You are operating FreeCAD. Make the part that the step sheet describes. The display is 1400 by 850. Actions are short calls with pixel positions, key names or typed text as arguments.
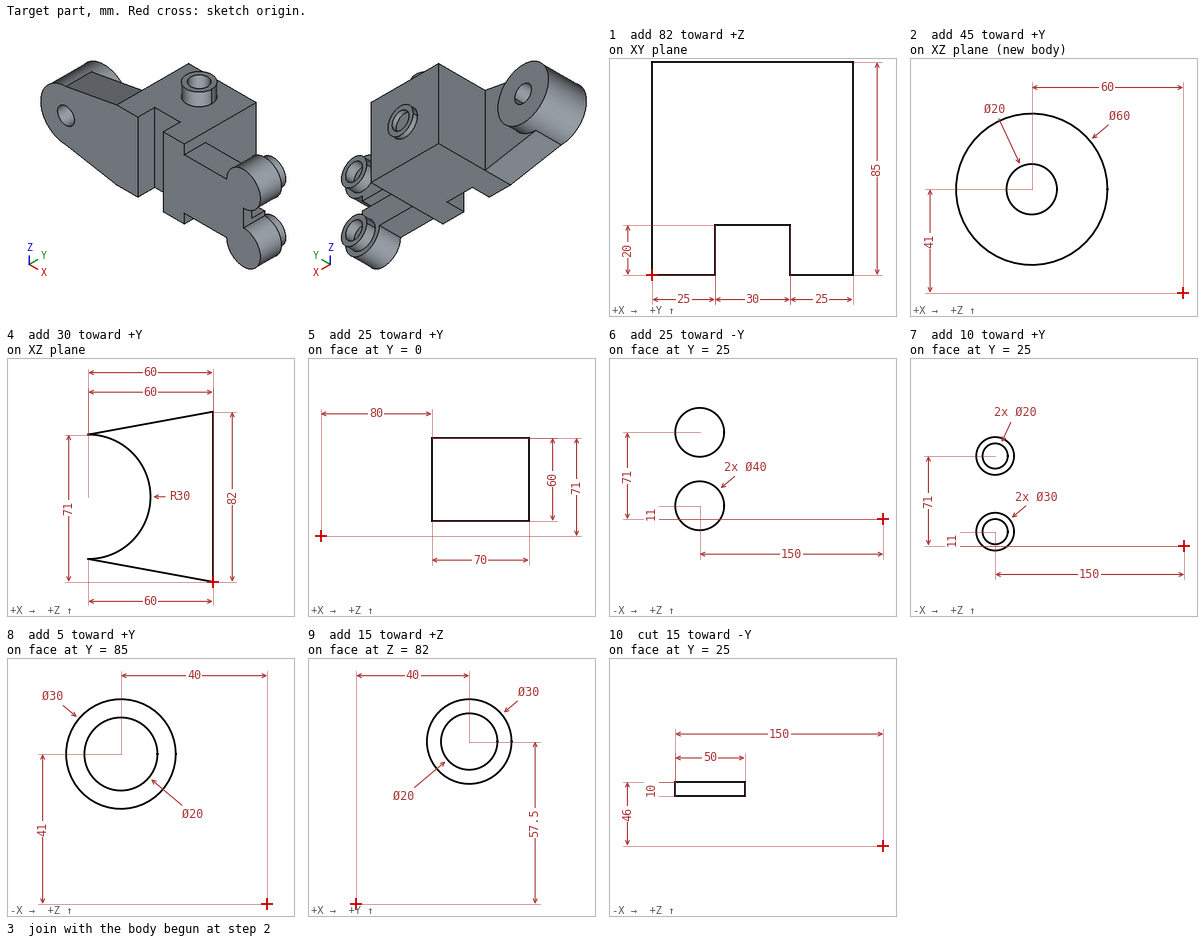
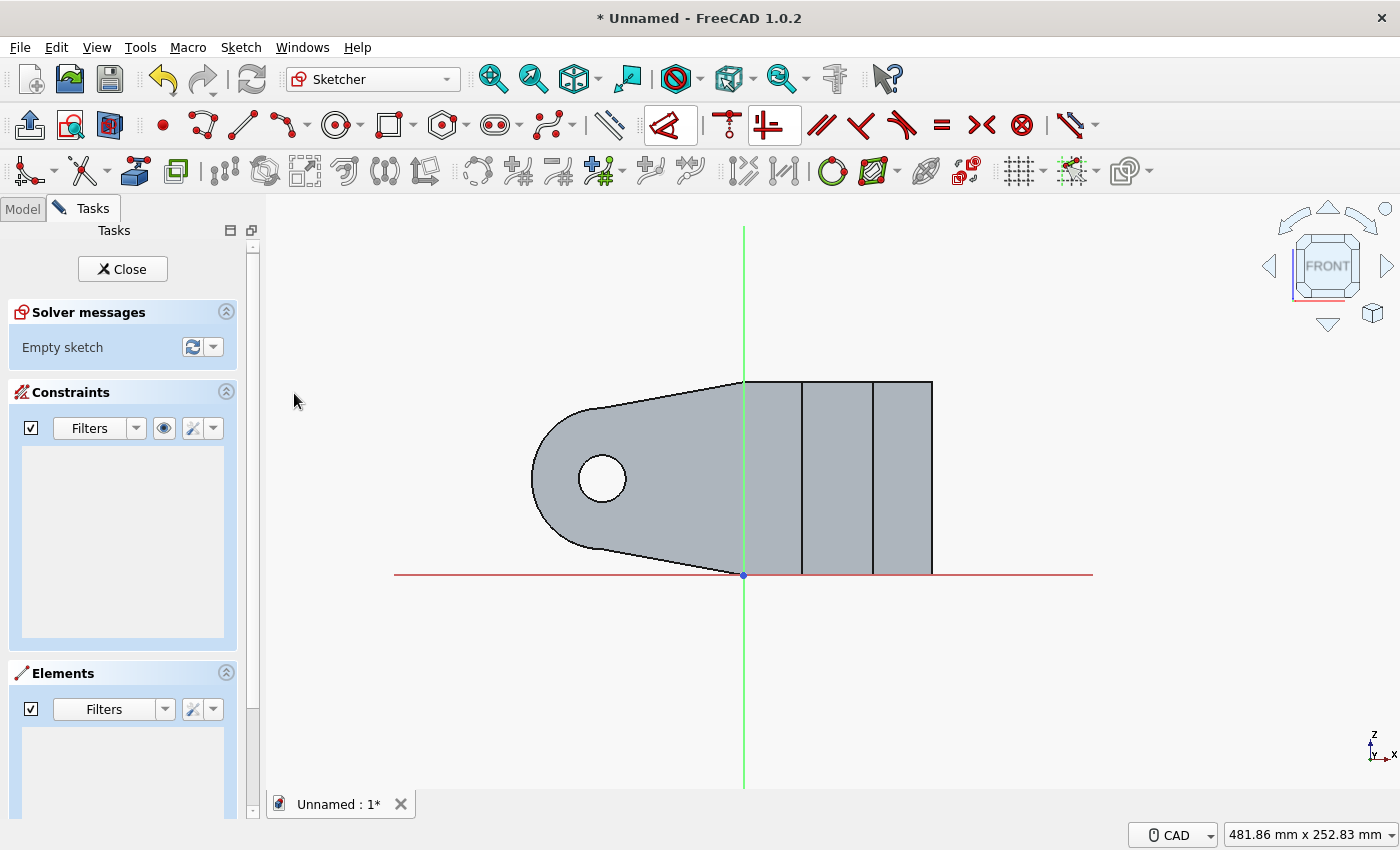
scroll(1109, 492, up, 3)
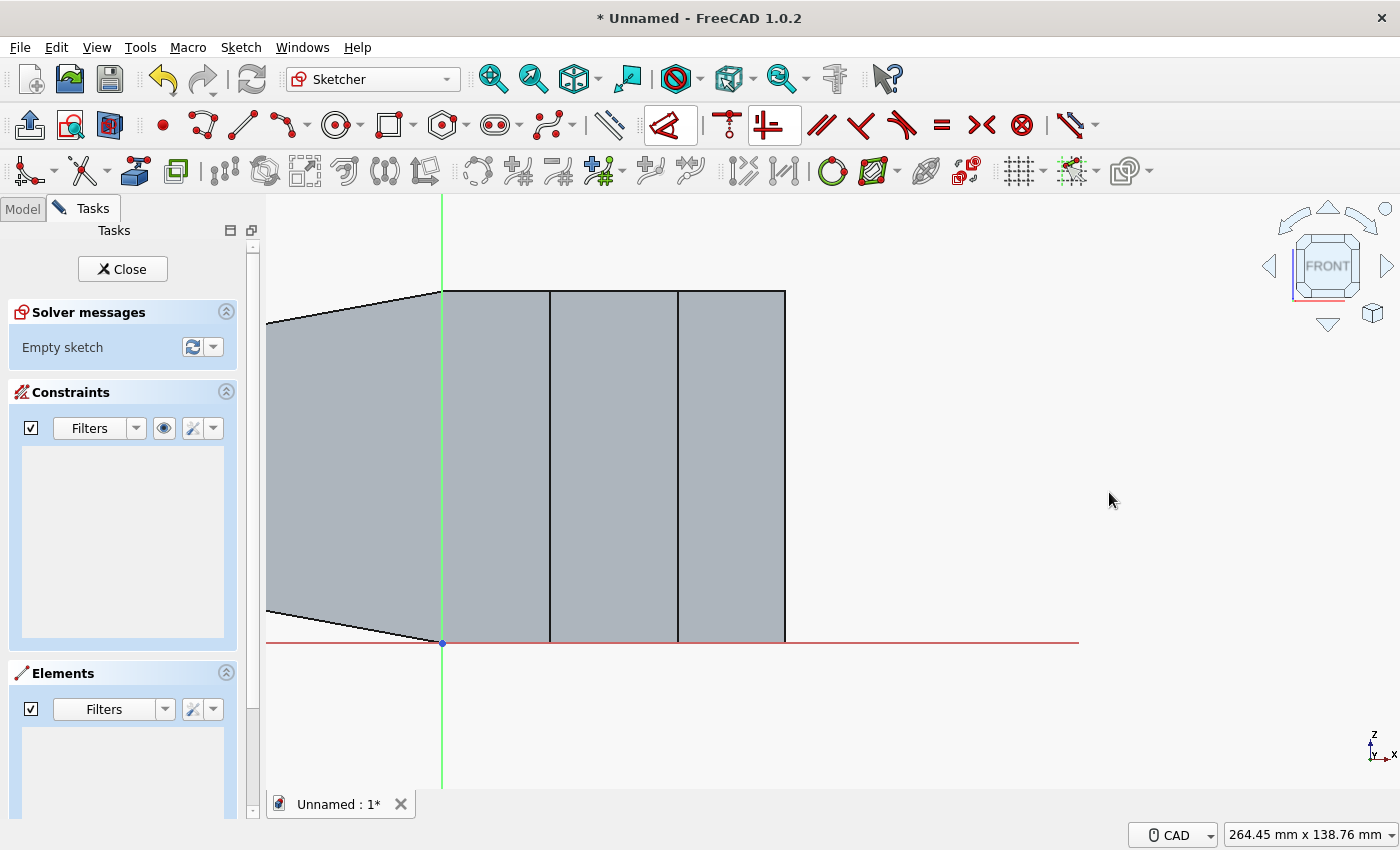
click(390, 126)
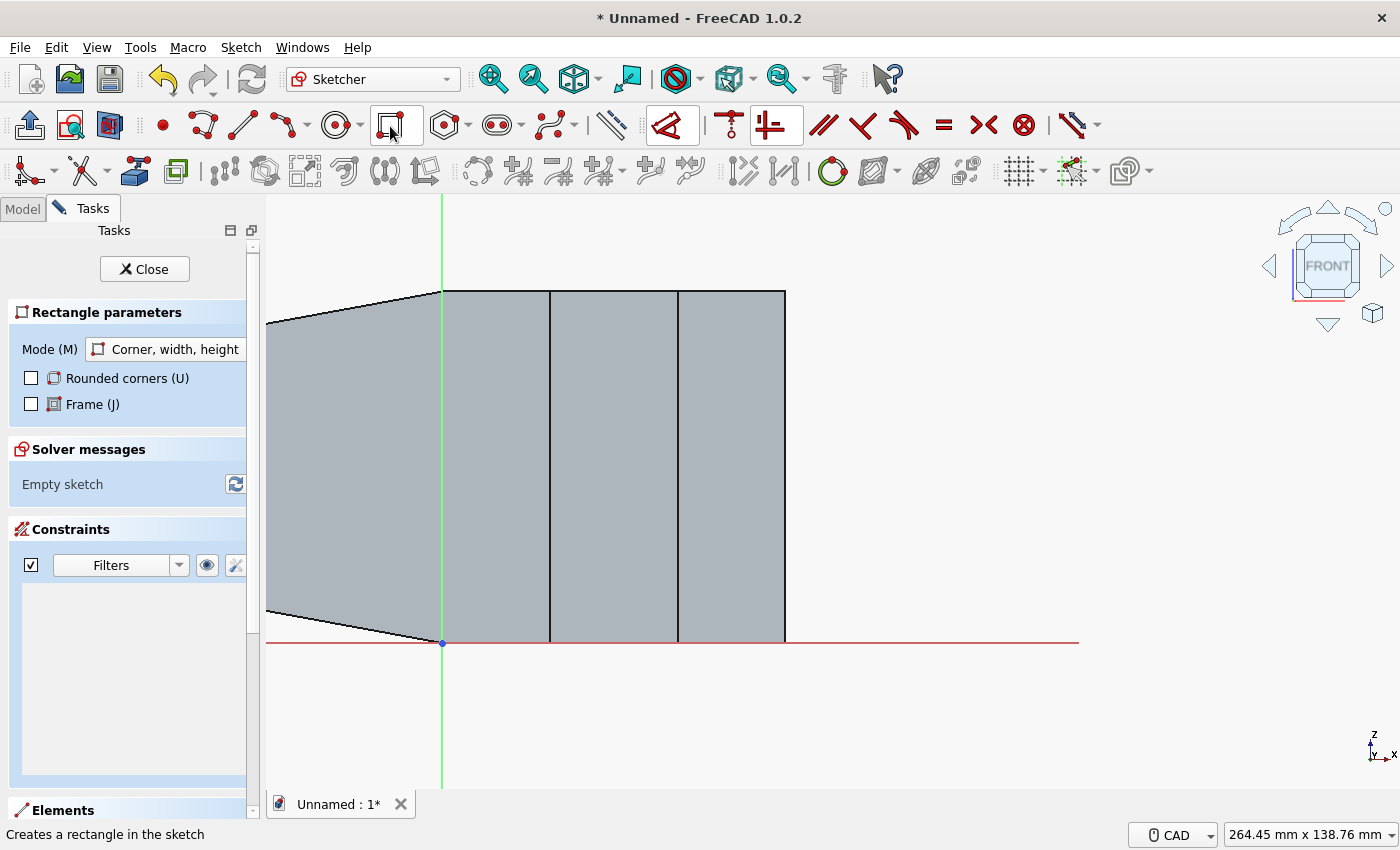
click(785, 339)
click(1086, 596)
key(Escape)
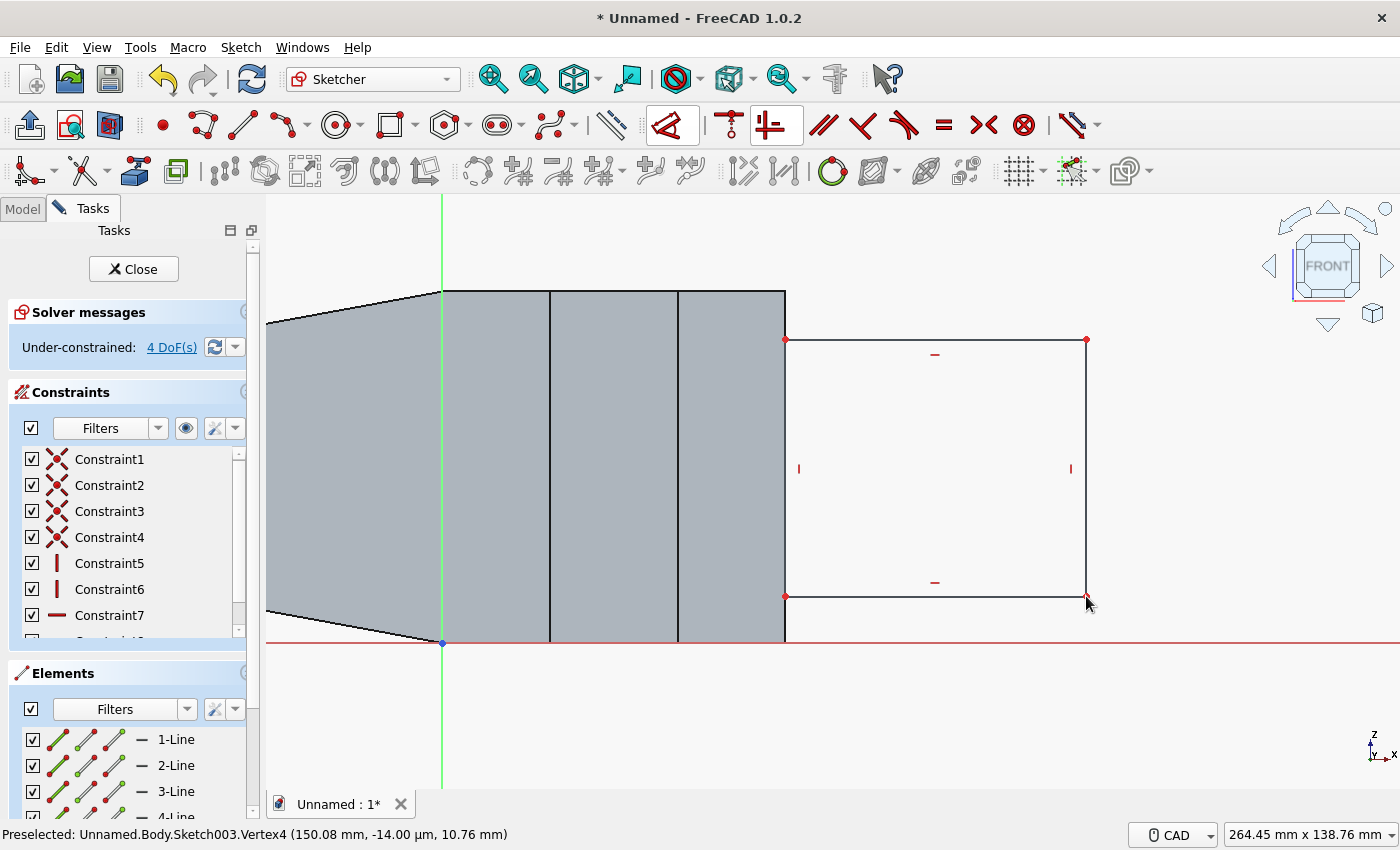
click(785, 417)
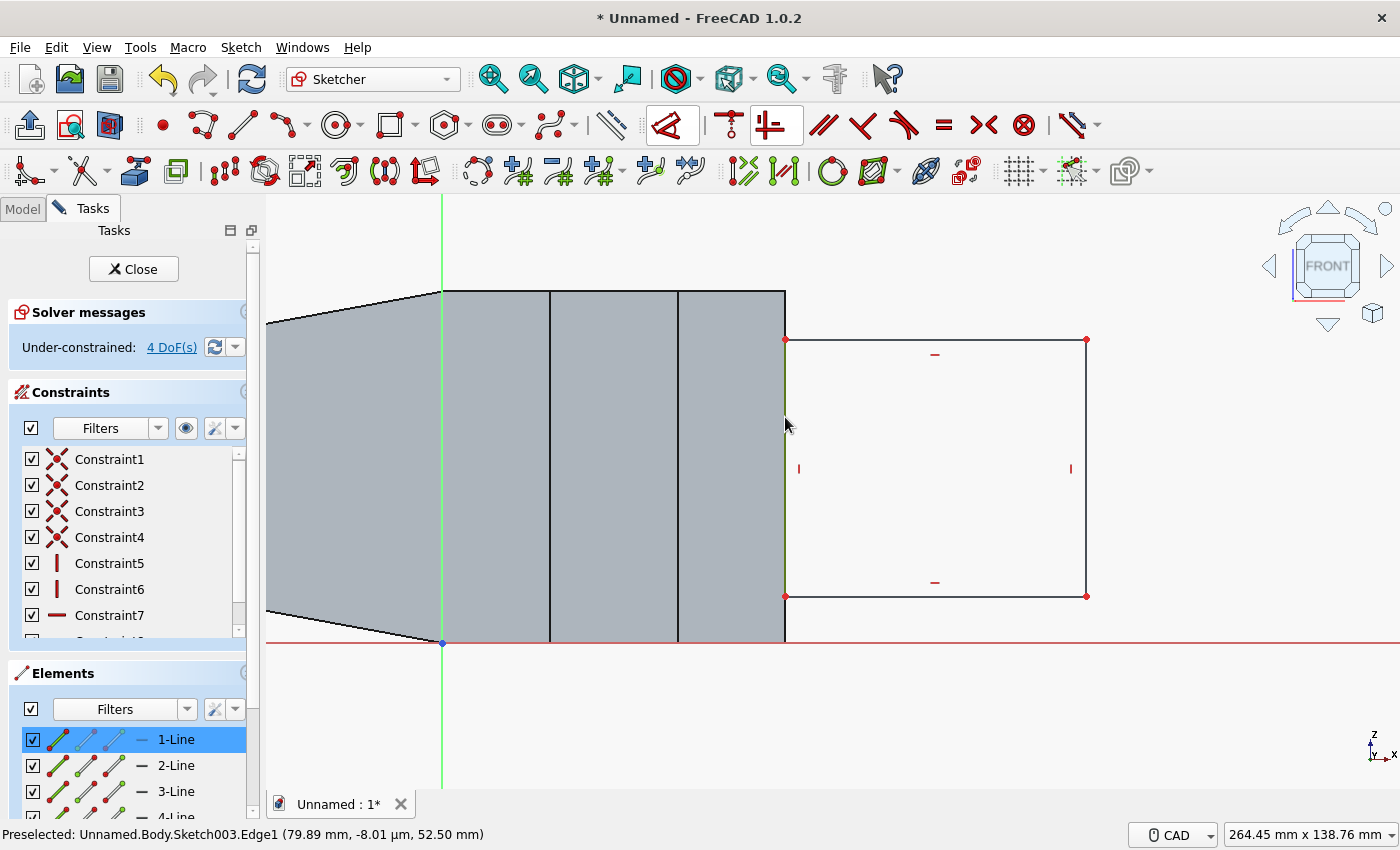
key(i)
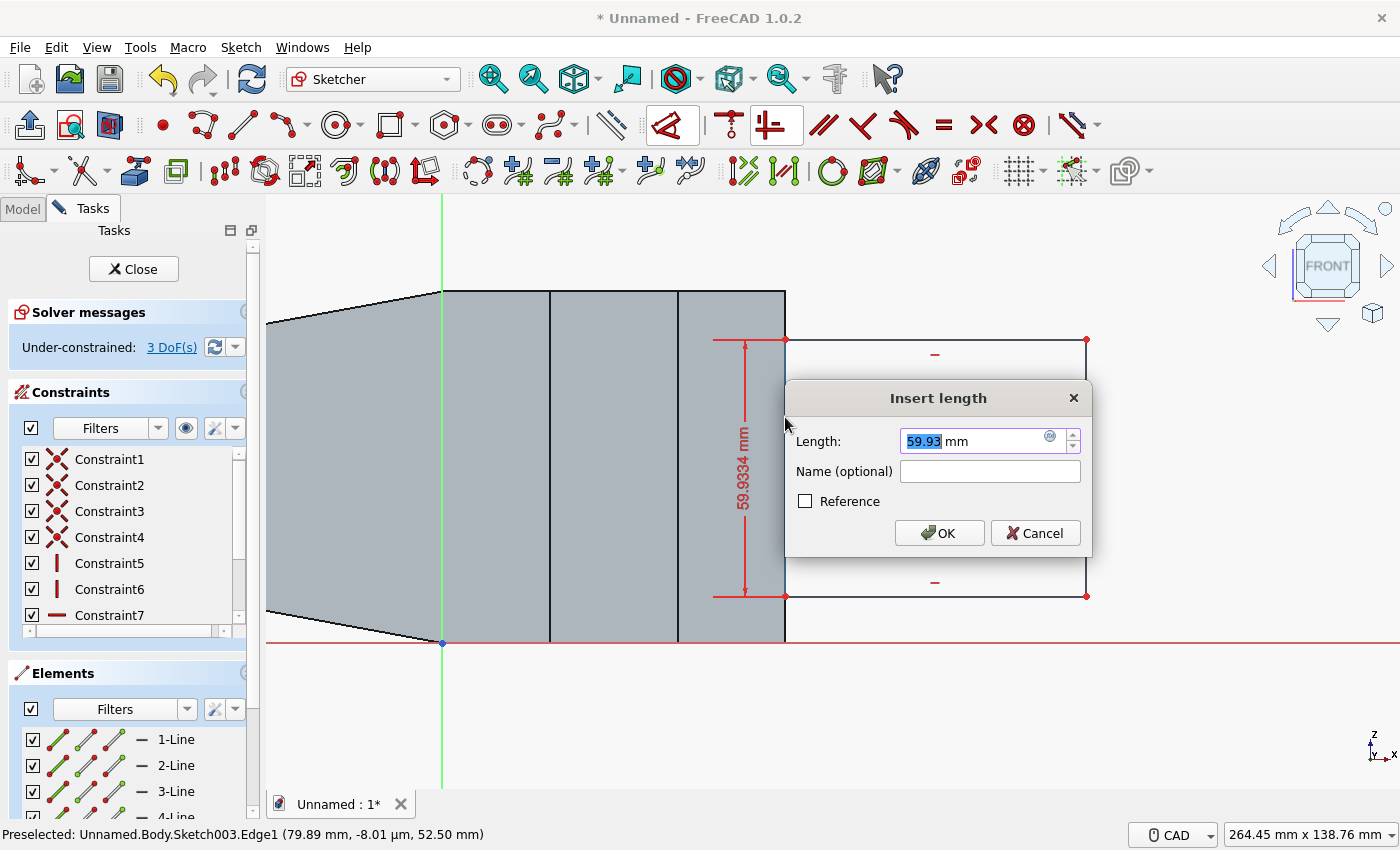
text(60)
key(Return)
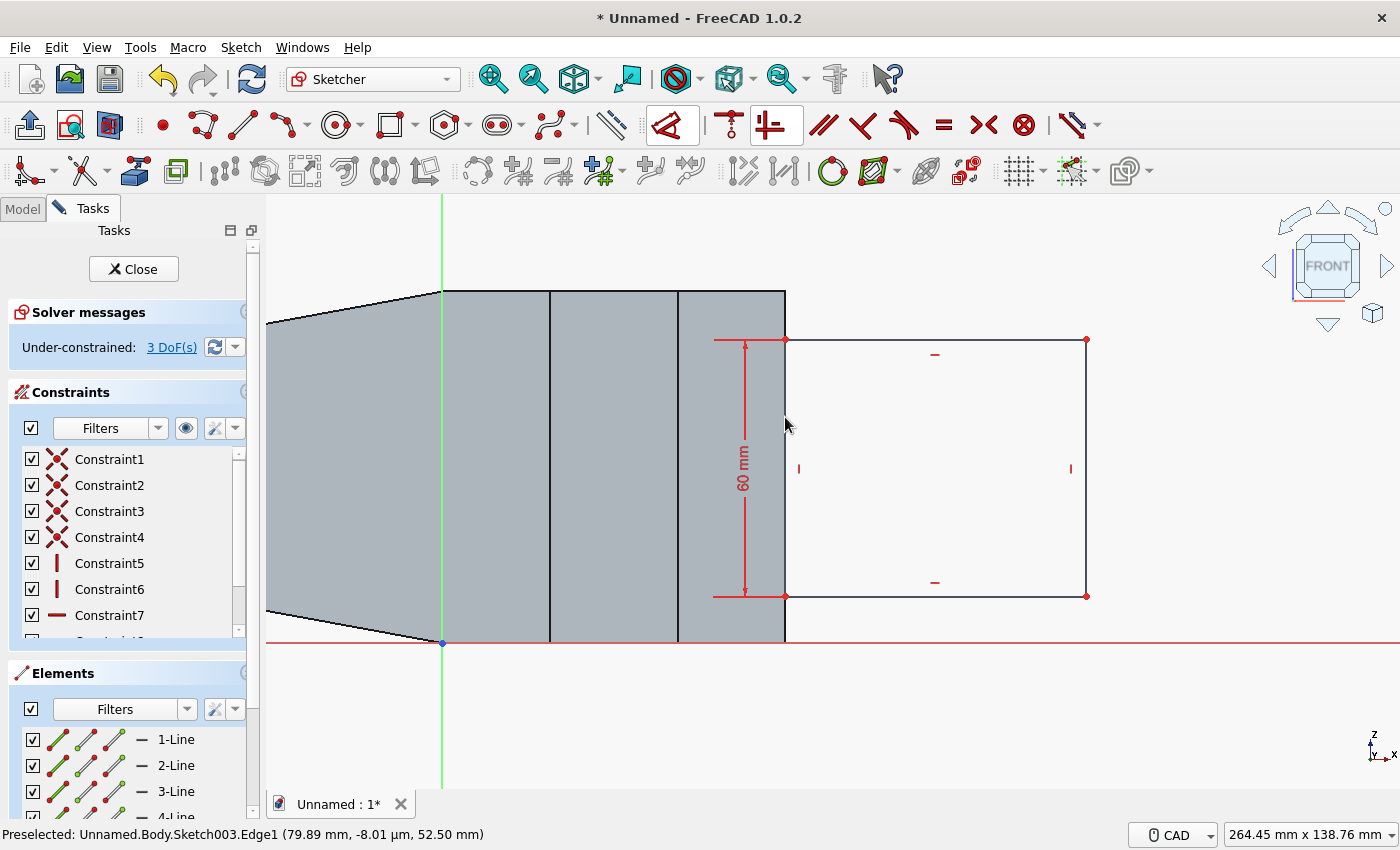
click(875, 597)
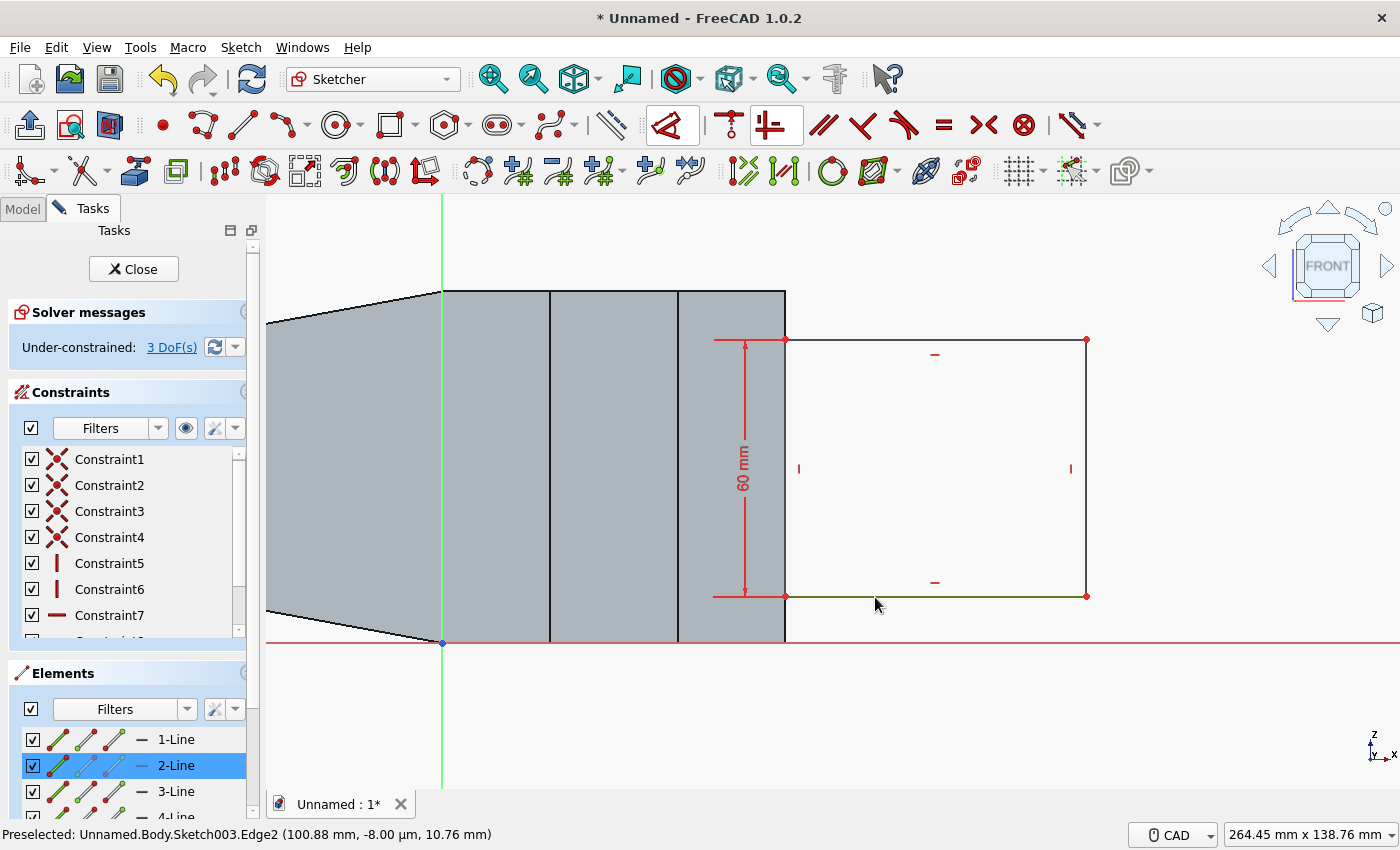
click(694, 126)